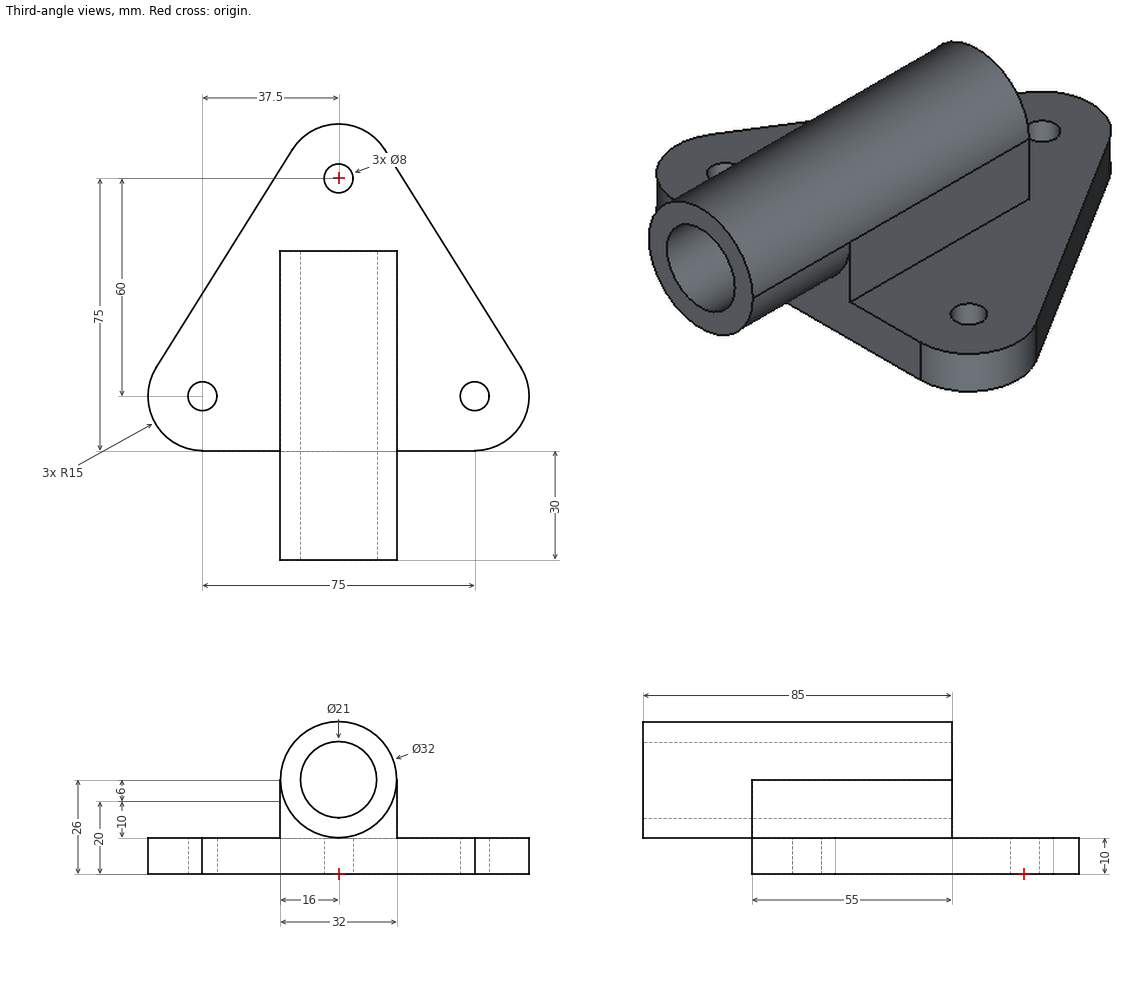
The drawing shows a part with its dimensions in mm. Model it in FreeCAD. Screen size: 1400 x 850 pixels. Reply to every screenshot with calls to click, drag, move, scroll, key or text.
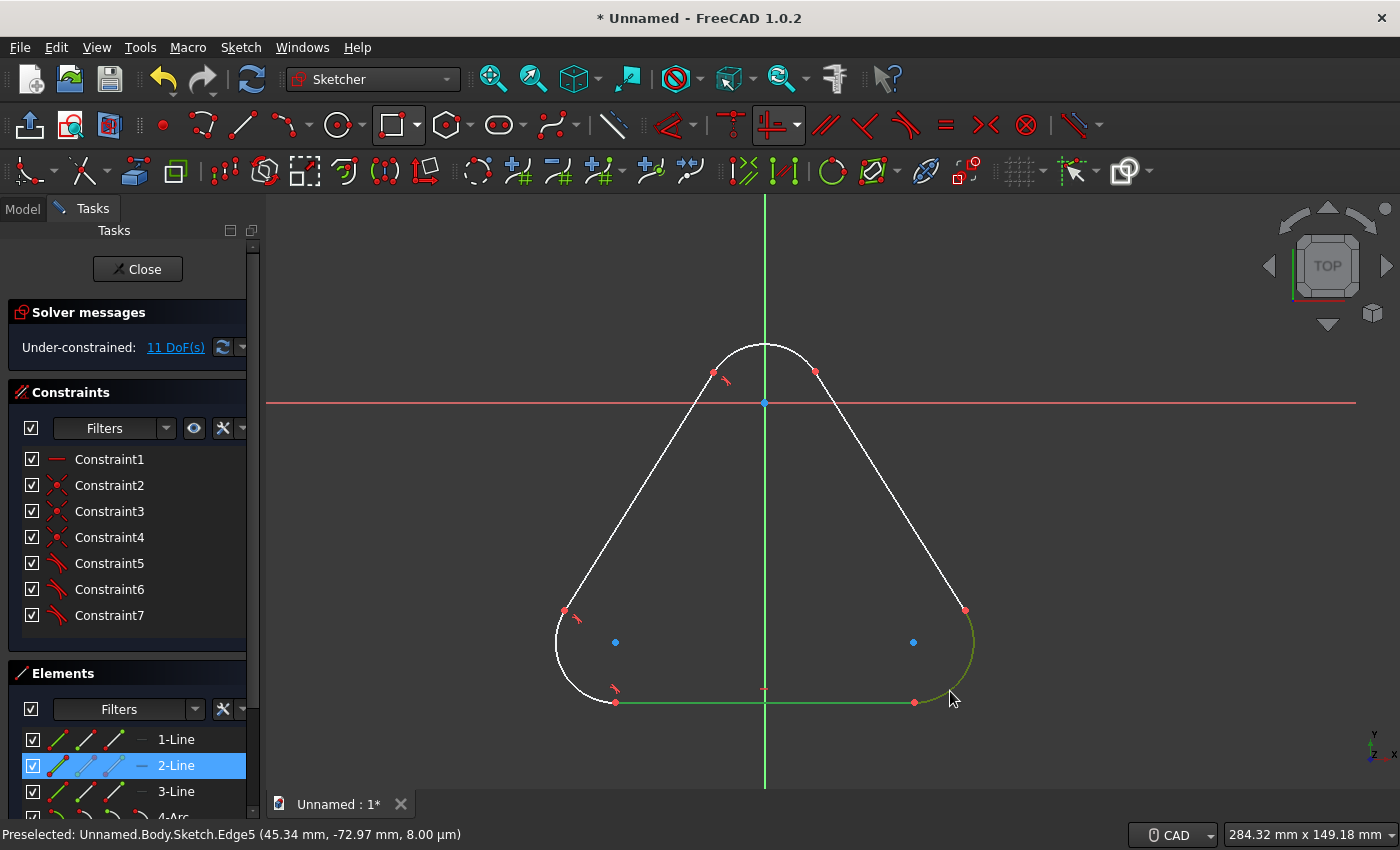
click(906, 126)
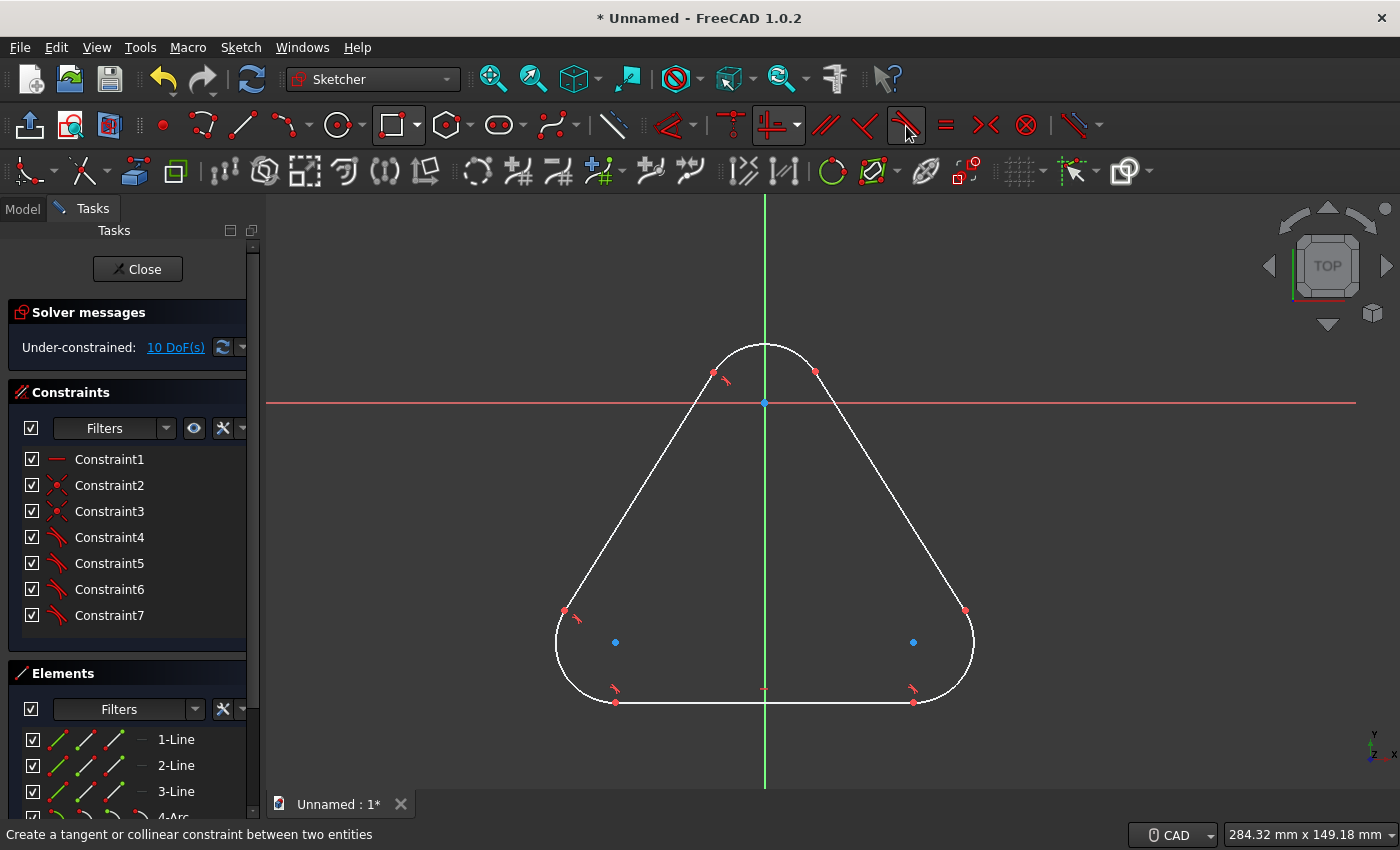
click(920, 539)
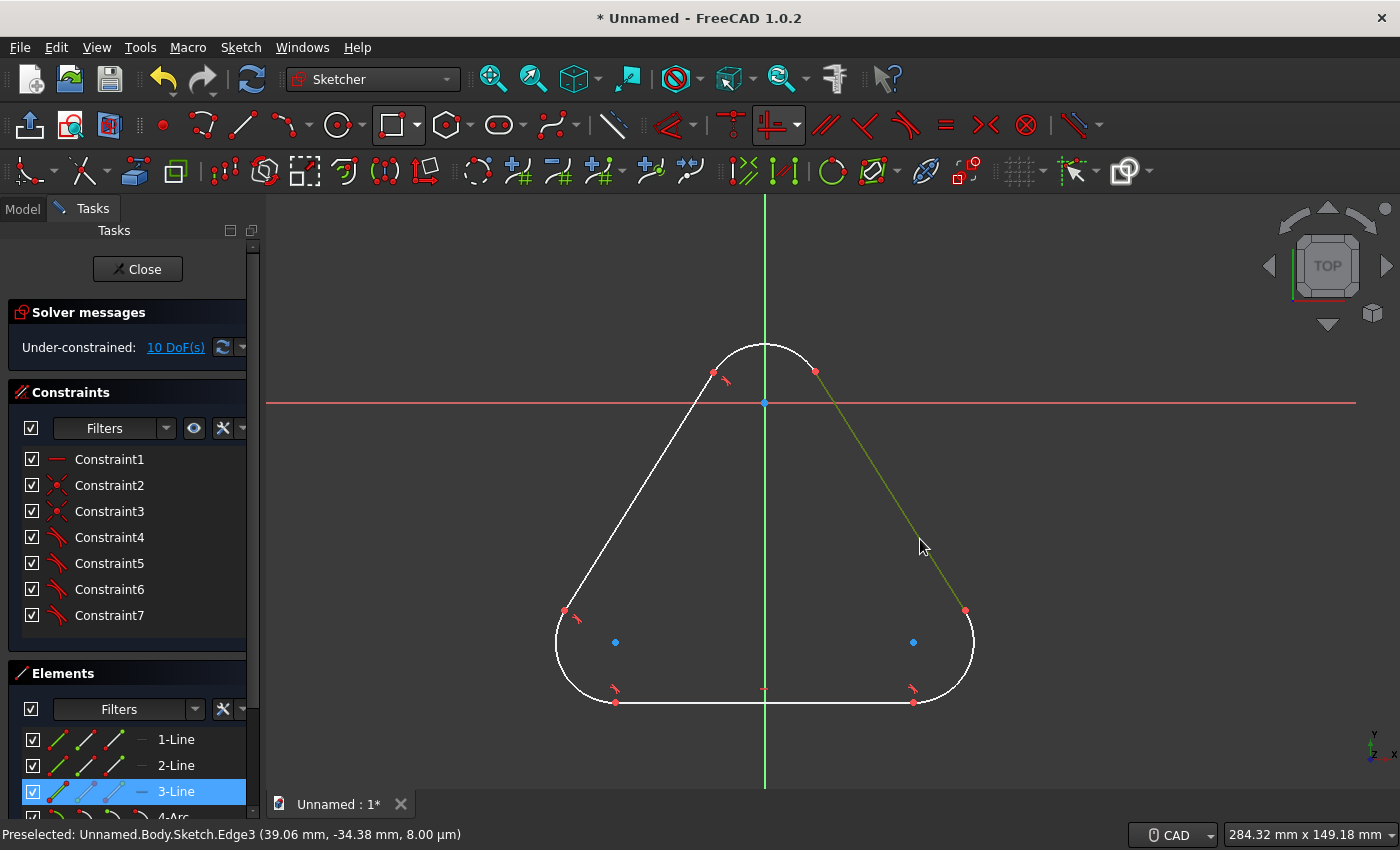
click(949, 691)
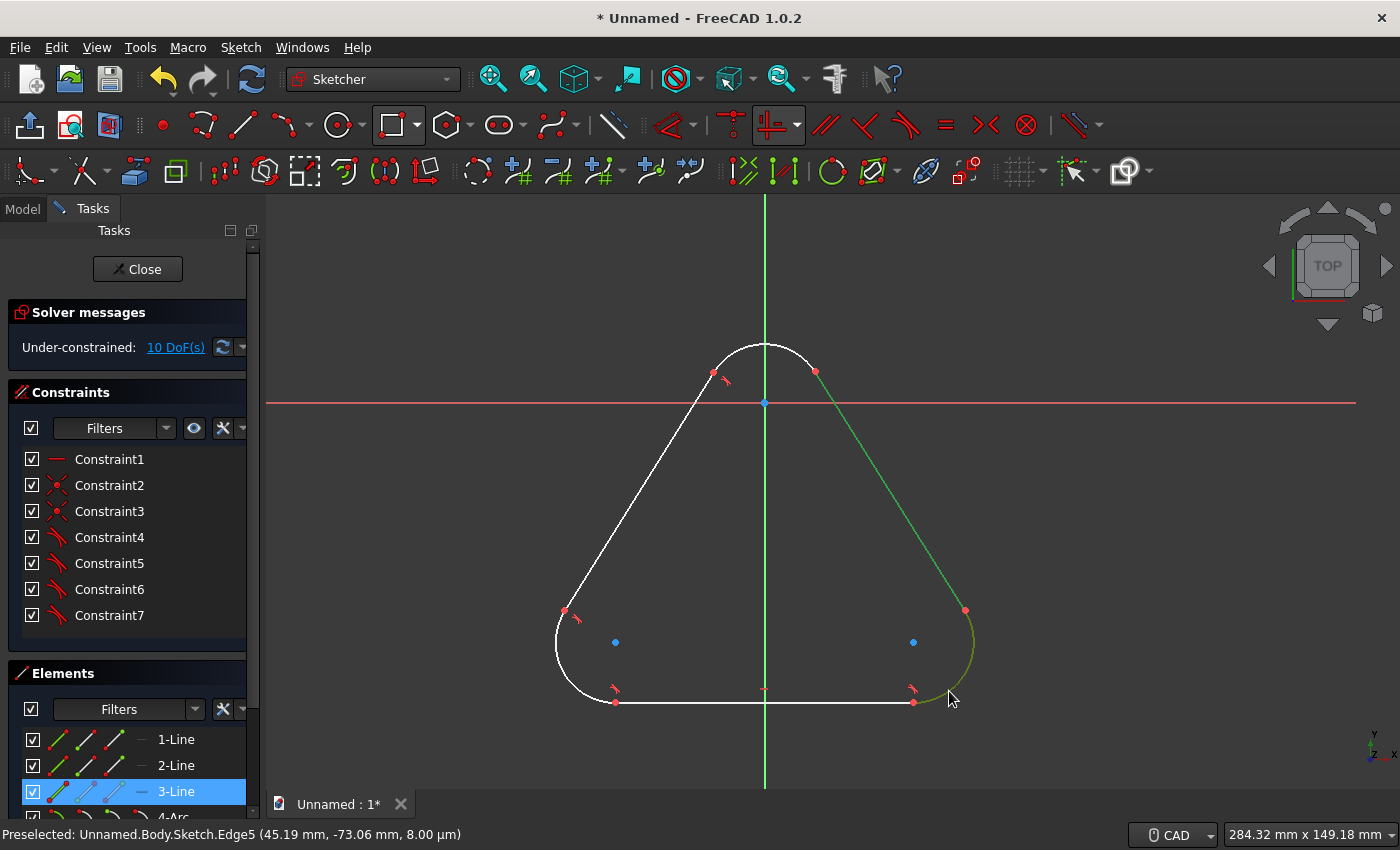
click(906, 126)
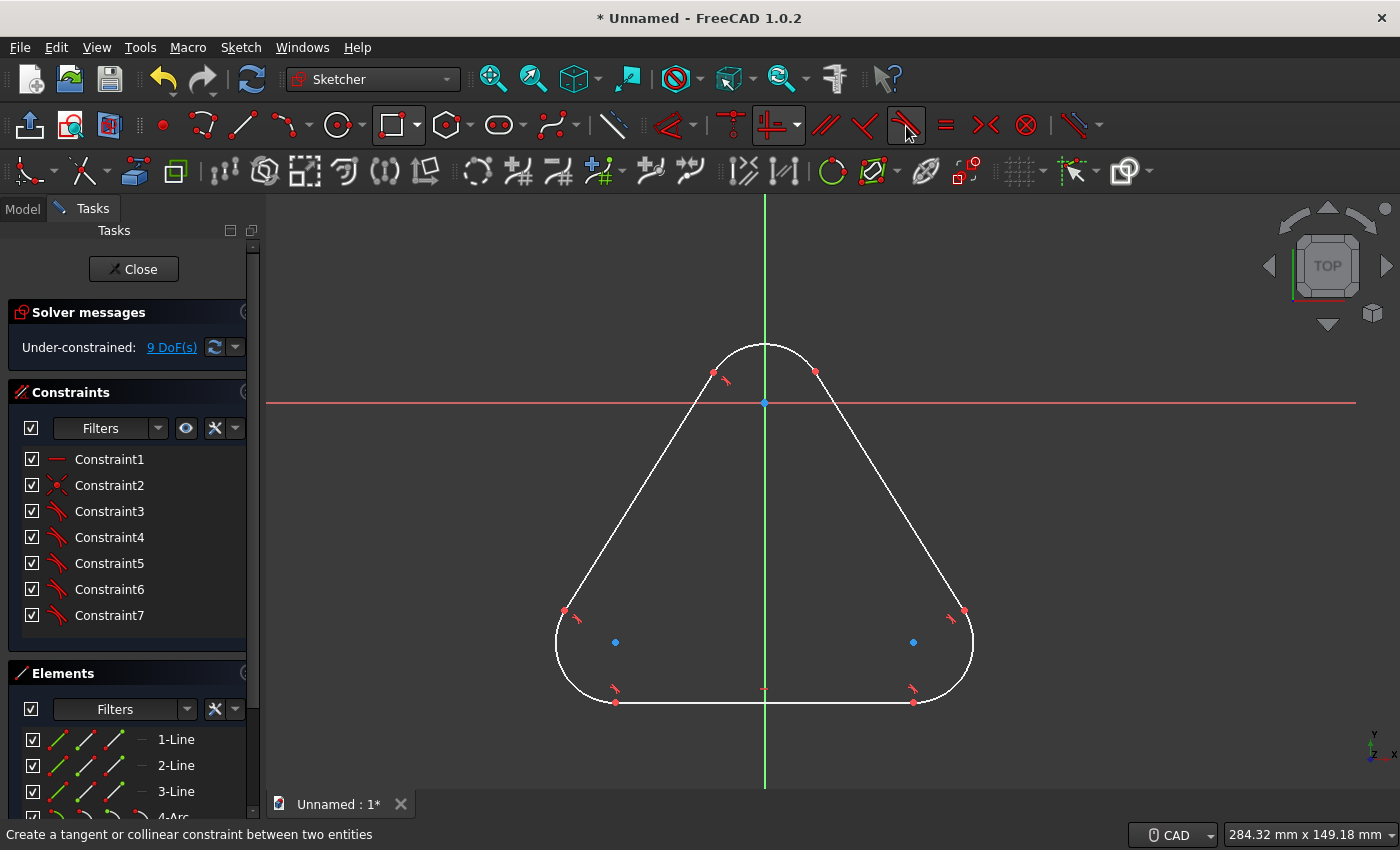
click(919, 539)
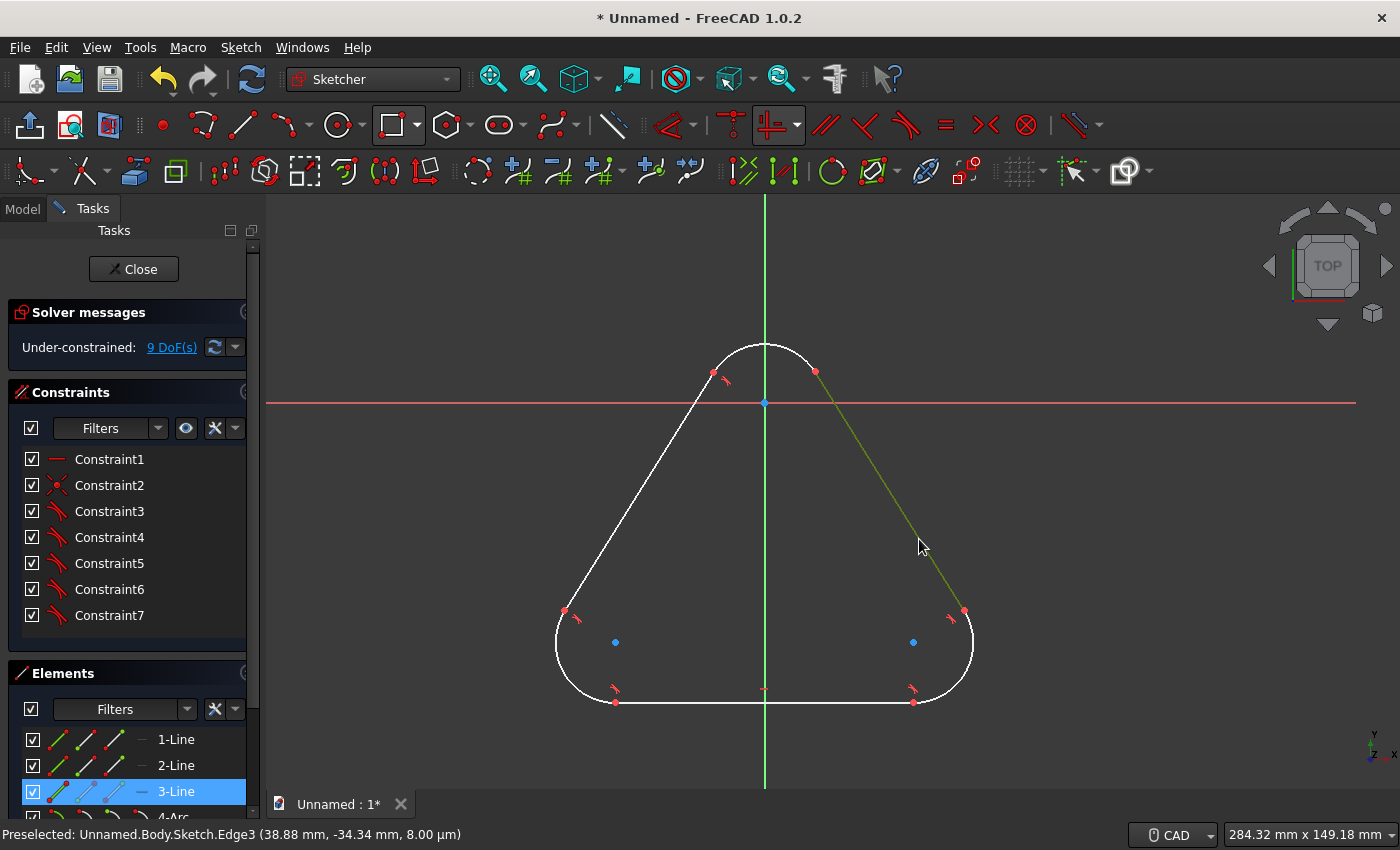
click(788, 349)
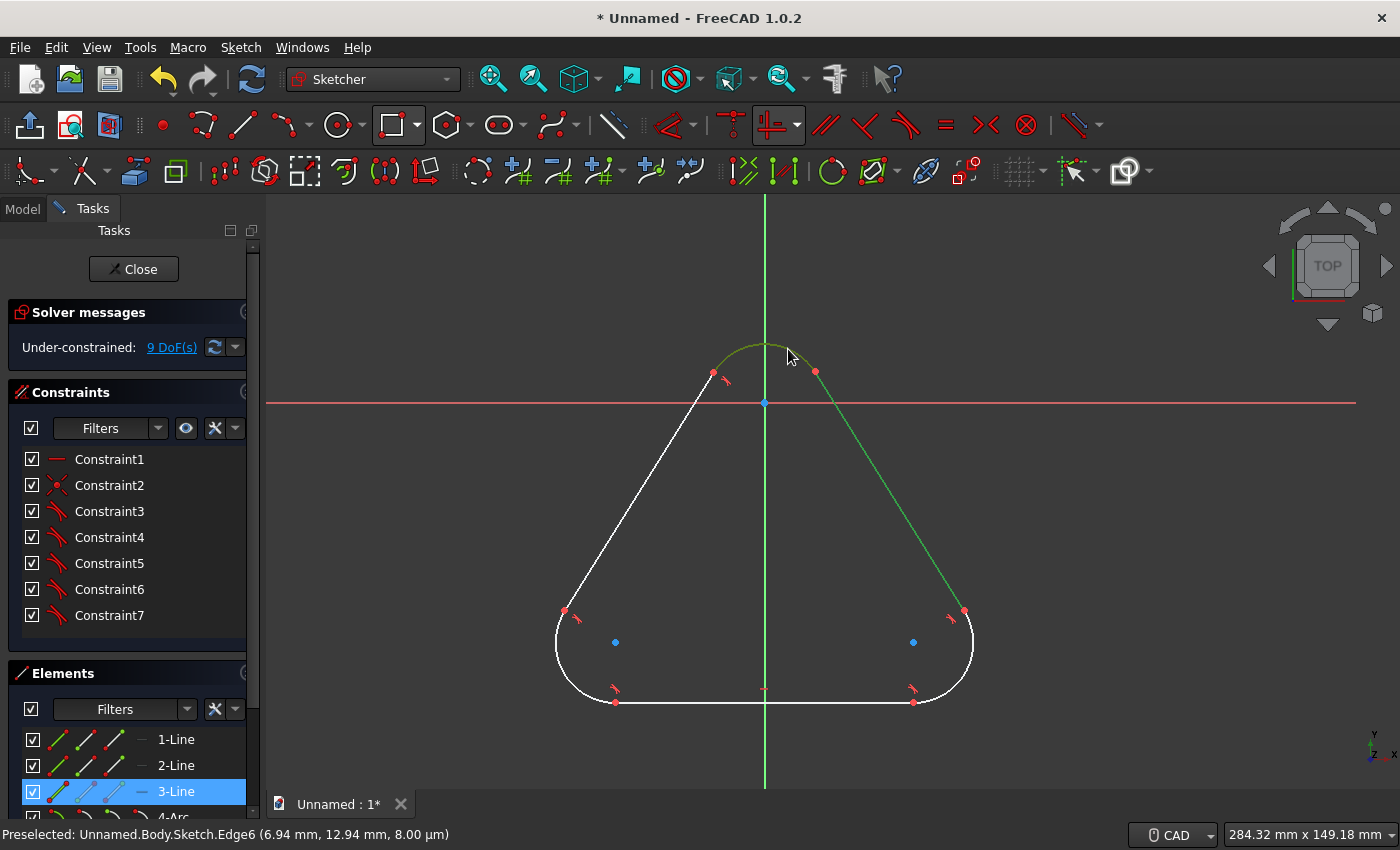
click(906, 126)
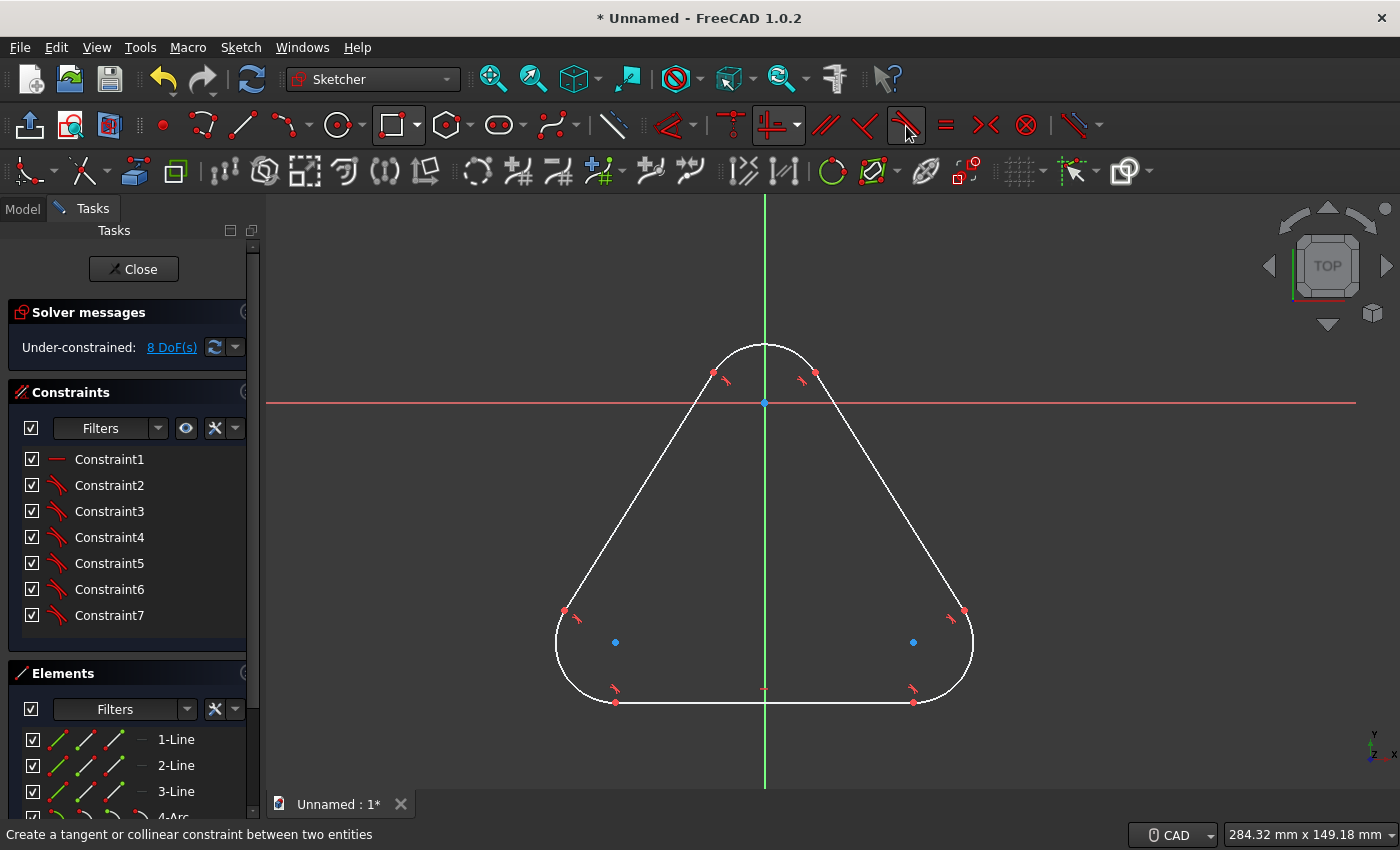
drag(754, 393, 775, 414)